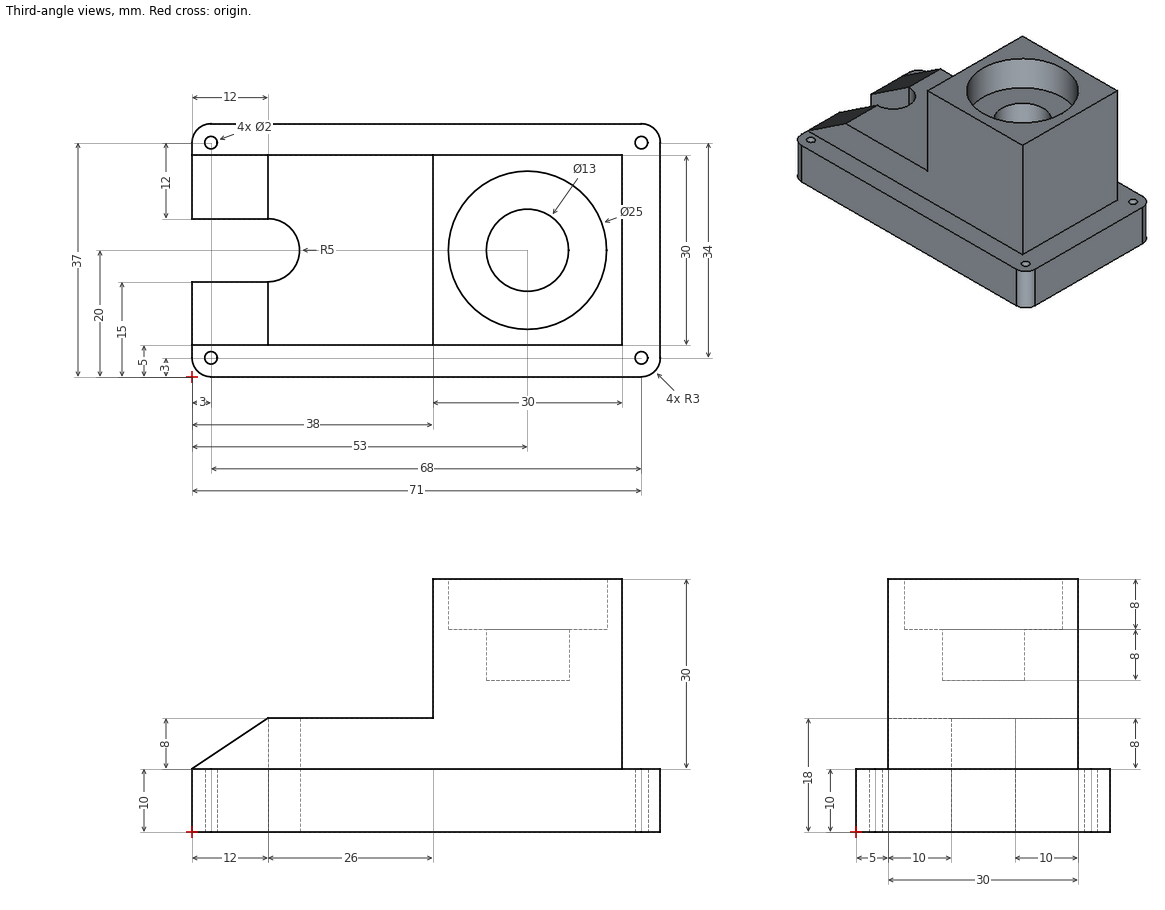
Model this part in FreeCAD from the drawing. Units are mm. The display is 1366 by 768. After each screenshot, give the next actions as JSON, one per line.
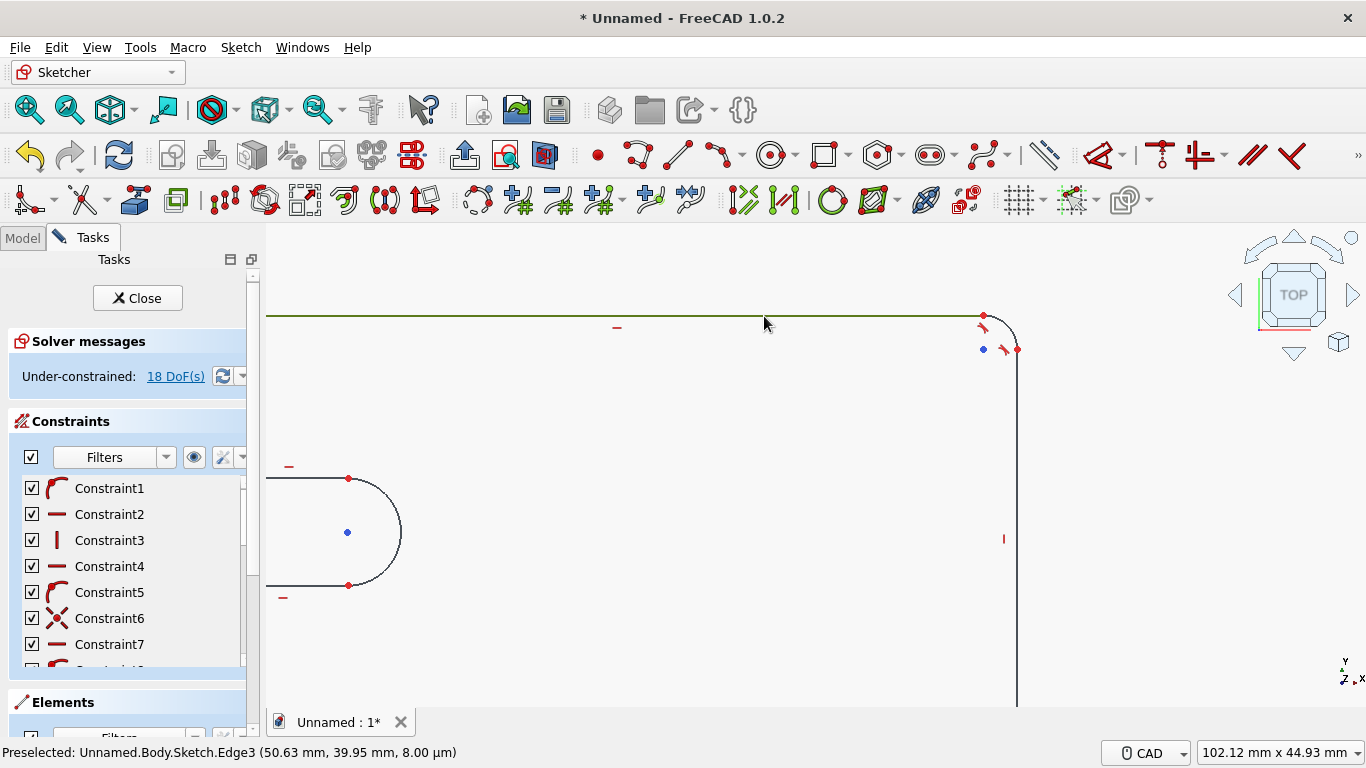
{"action": "scroll", "coordinate": [1013, 332], "scroll_direction": "down", "scroll_amount": 2}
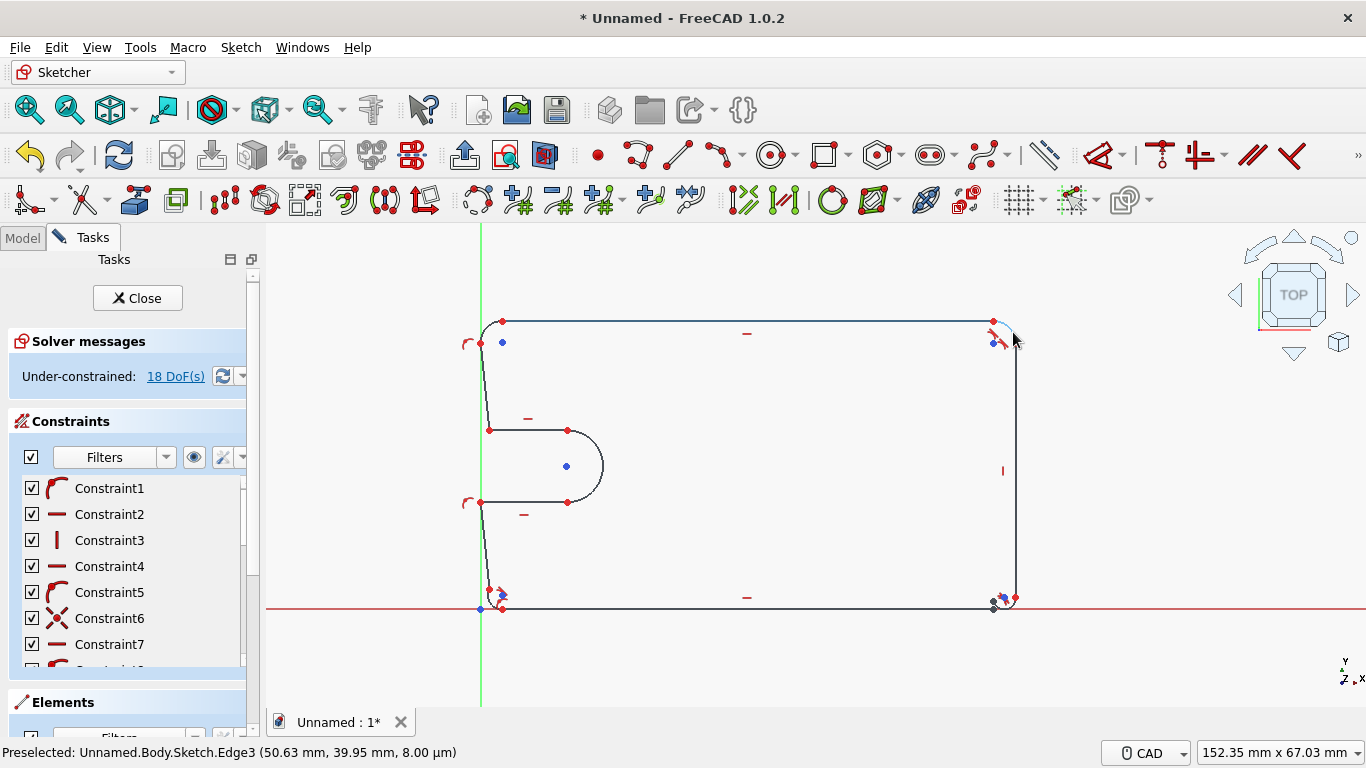
{"action": "scroll", "coordinate": [492, 323], "scroll_direction": "up", "scroll_amount": 2}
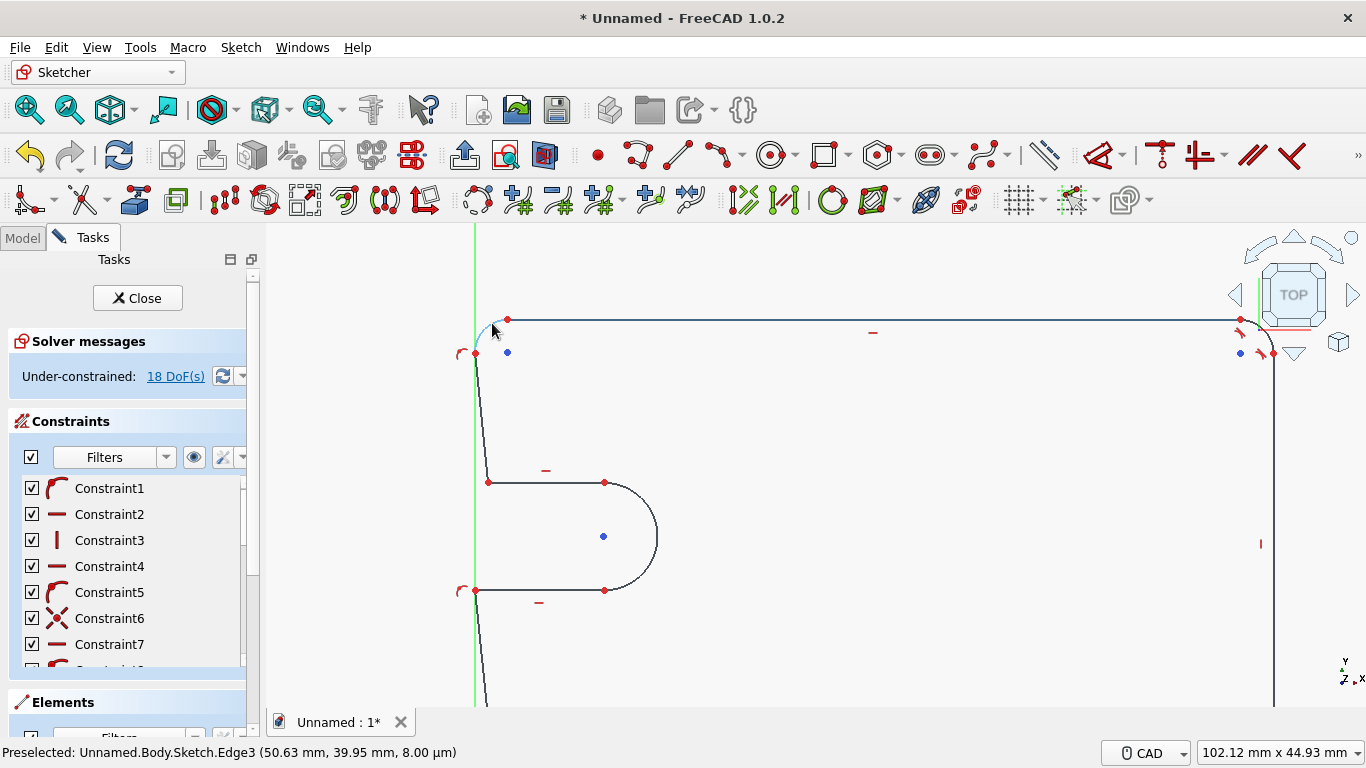
{"action": "left_click", "coordinate": [493, 324]}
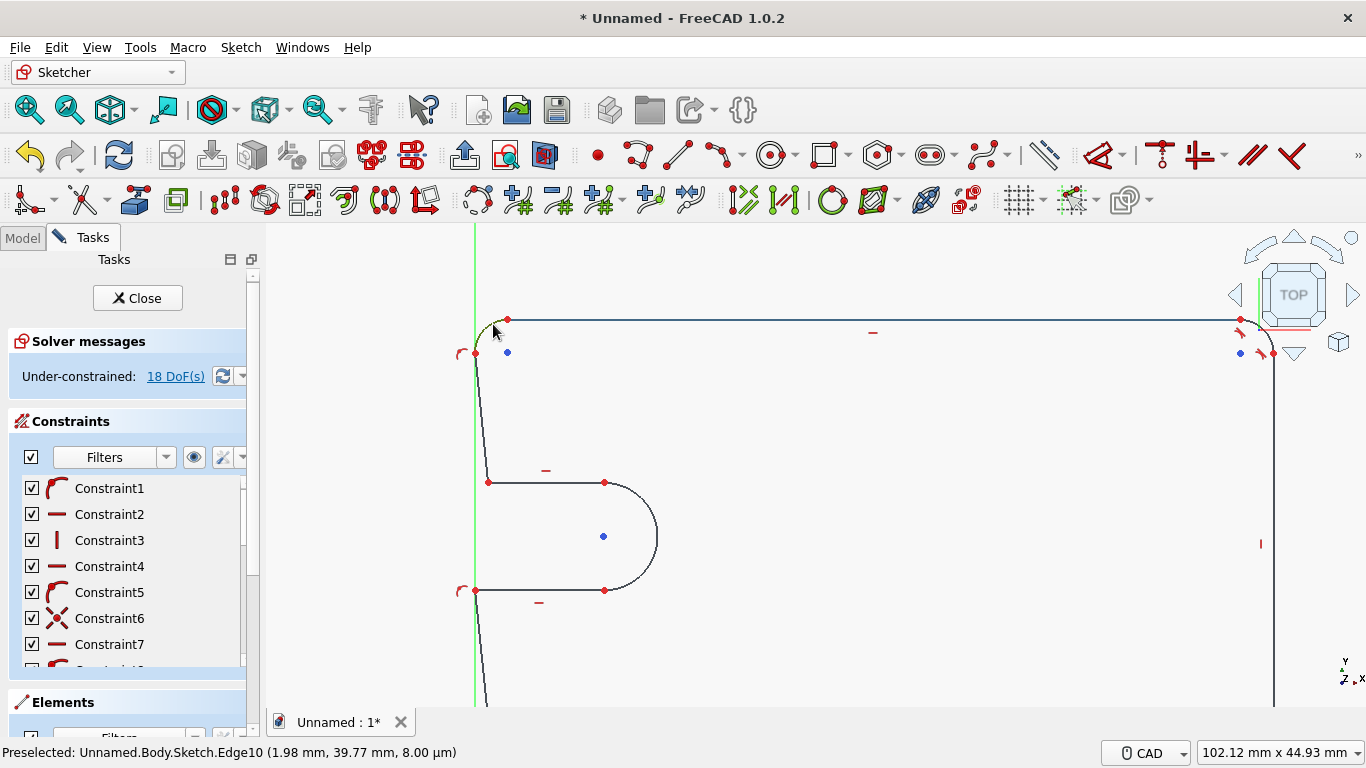
{"action": "key", "text": "t"}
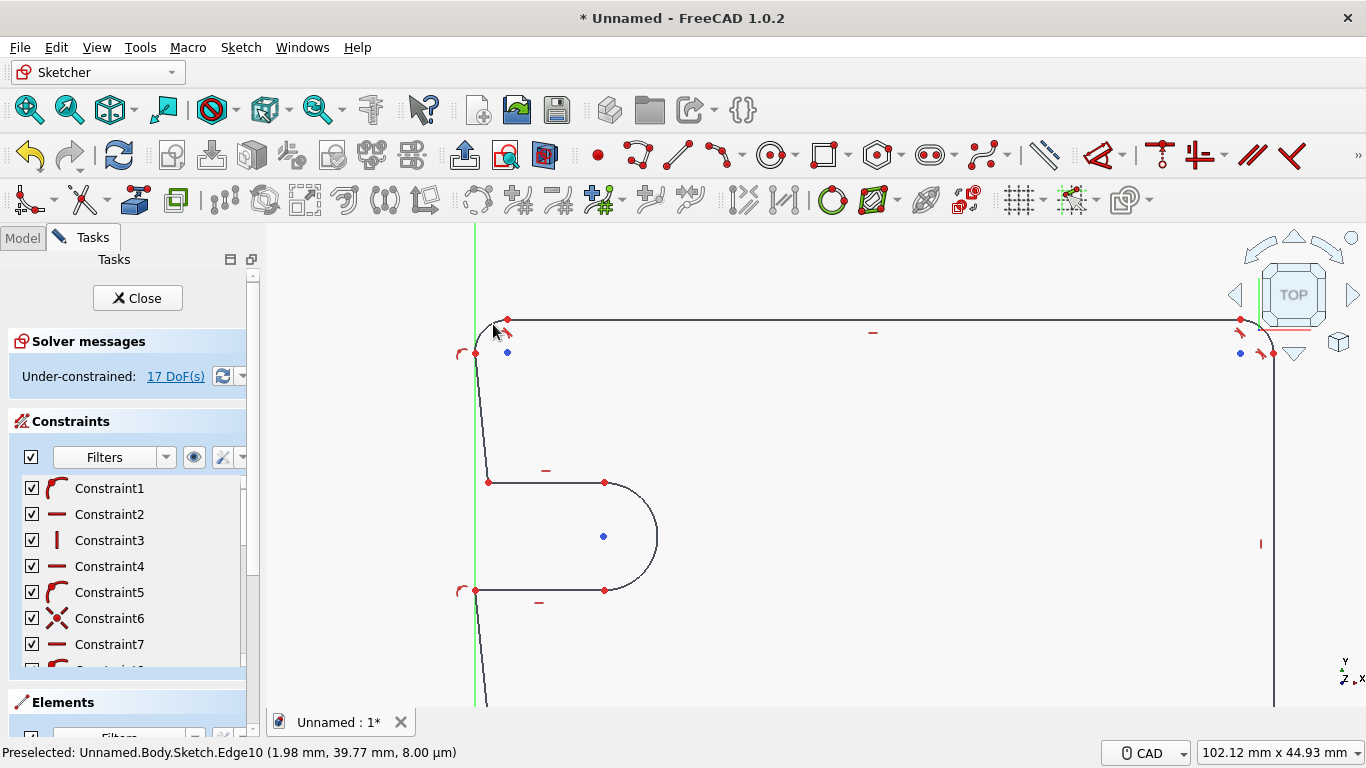
{"action": "left_click", "coordinate": [479, 392]}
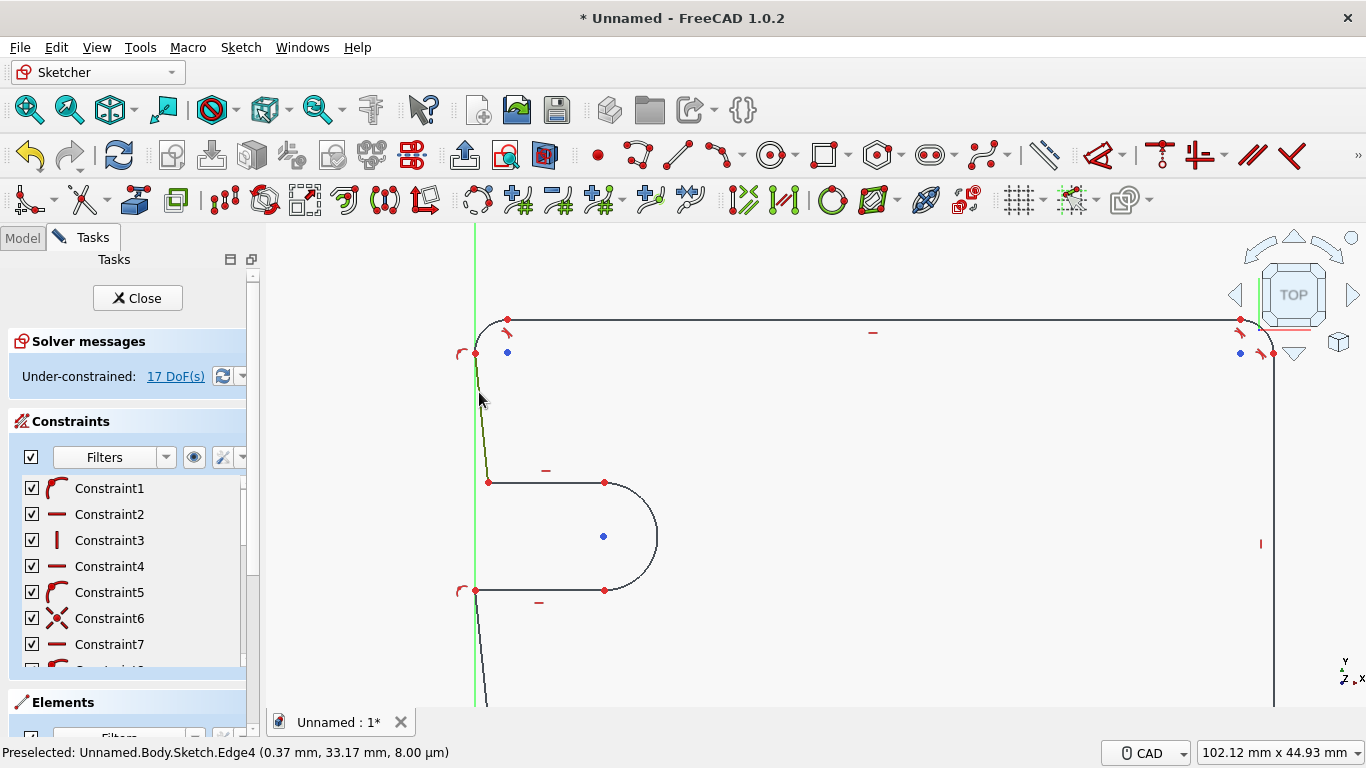
{"action": "left_click", "coordinate": [493, 324]}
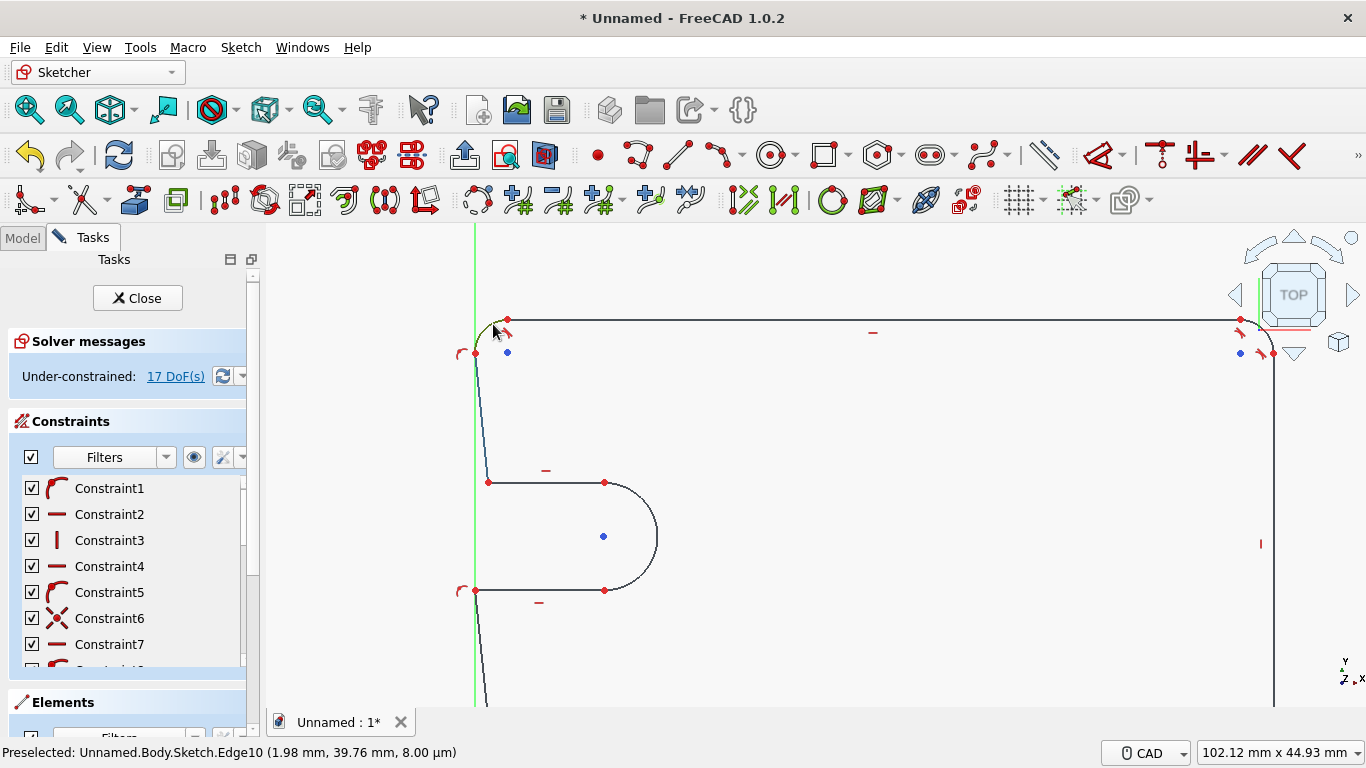
{"action": "key", "text": "t"}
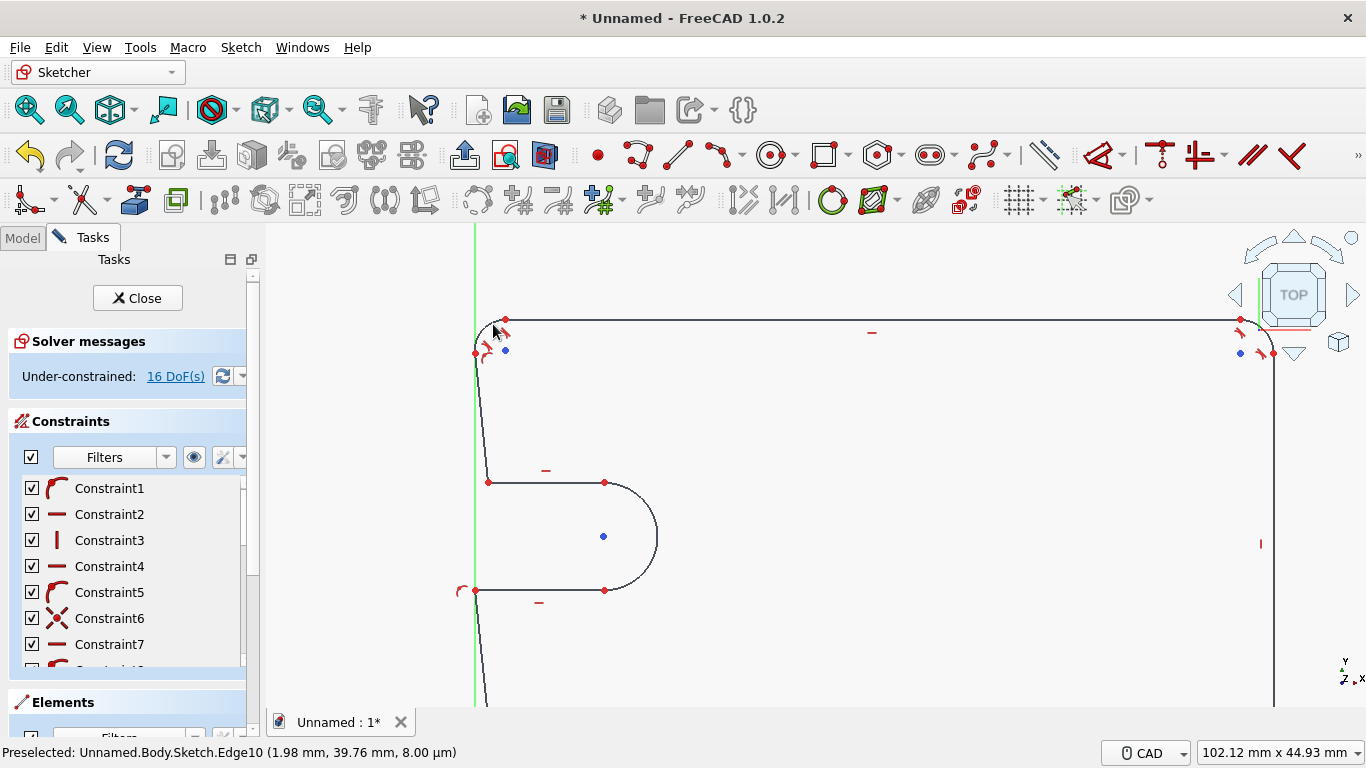
{"action": "left_click", "coordinate": [523, 483]}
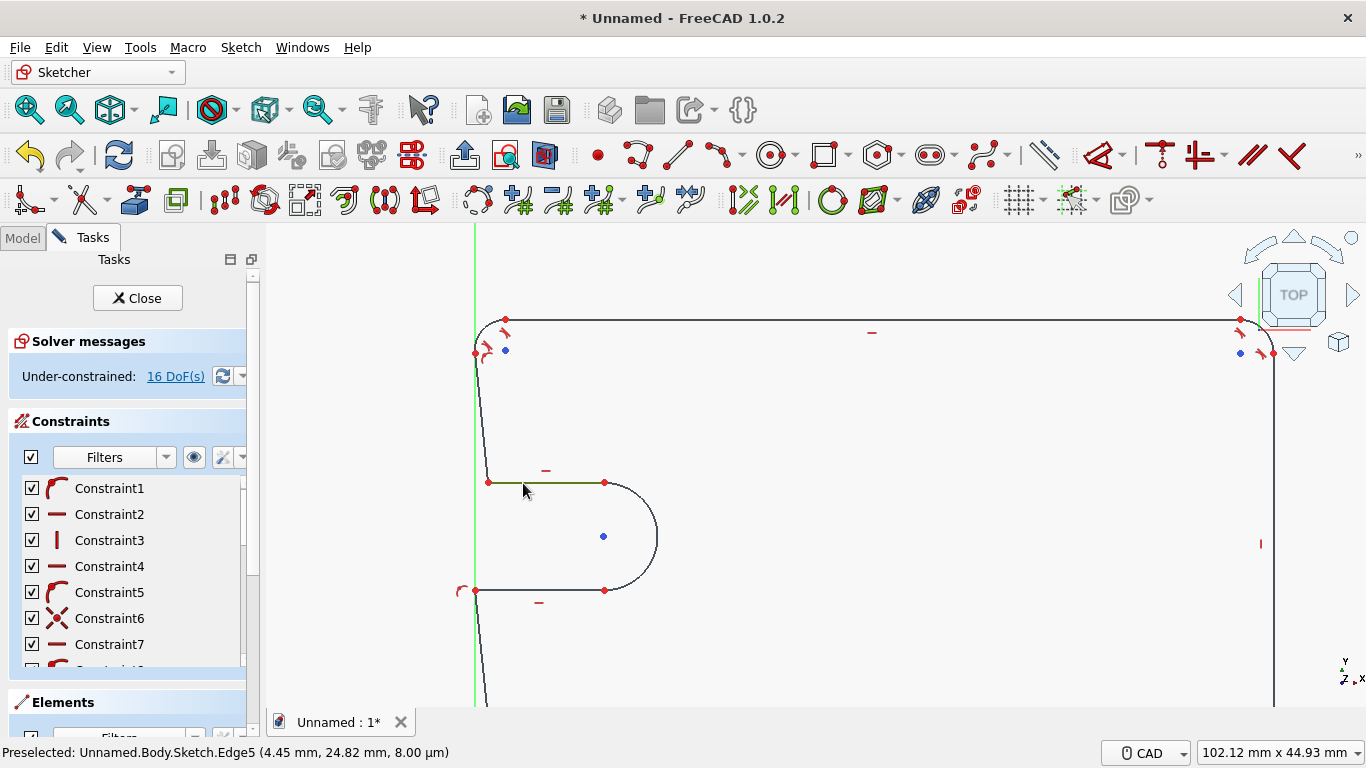
{"action": "left_click", "coordinate": [647, 568]}